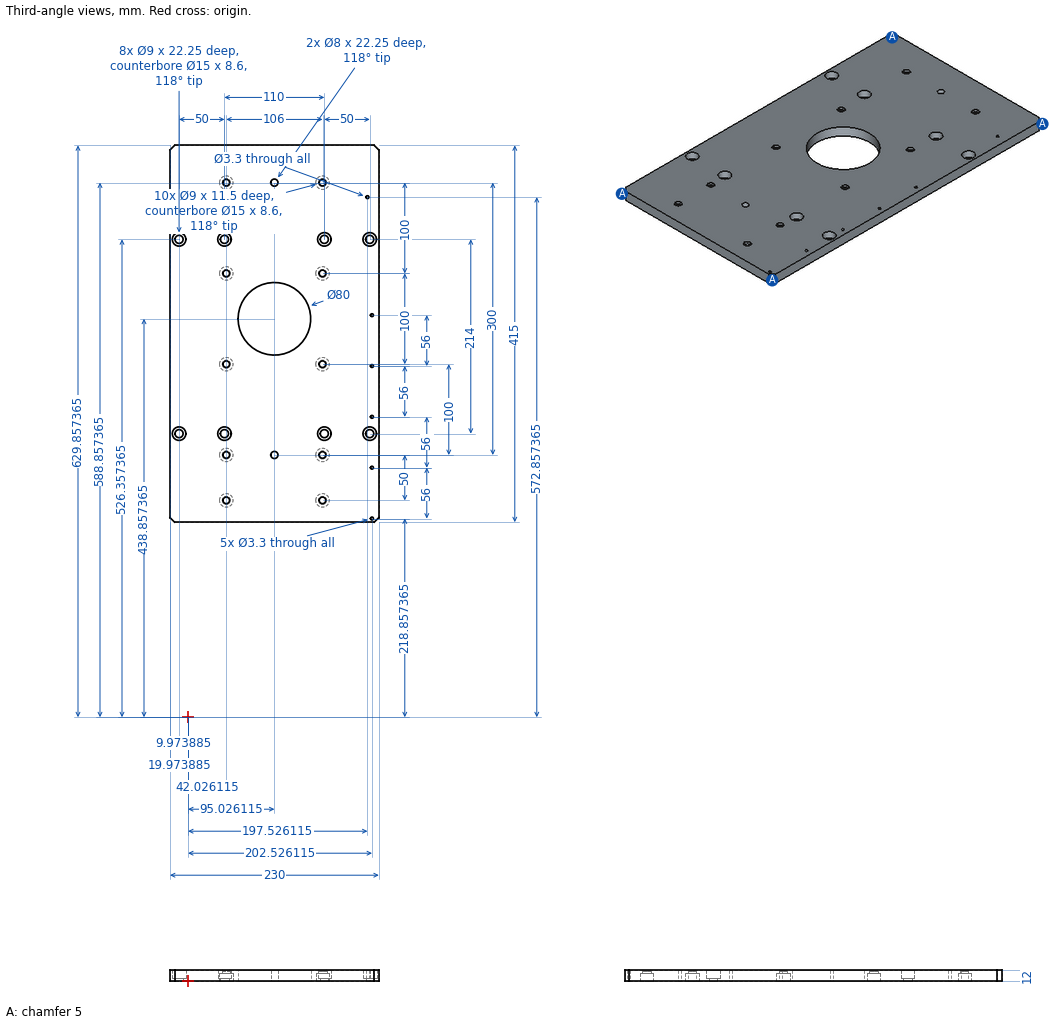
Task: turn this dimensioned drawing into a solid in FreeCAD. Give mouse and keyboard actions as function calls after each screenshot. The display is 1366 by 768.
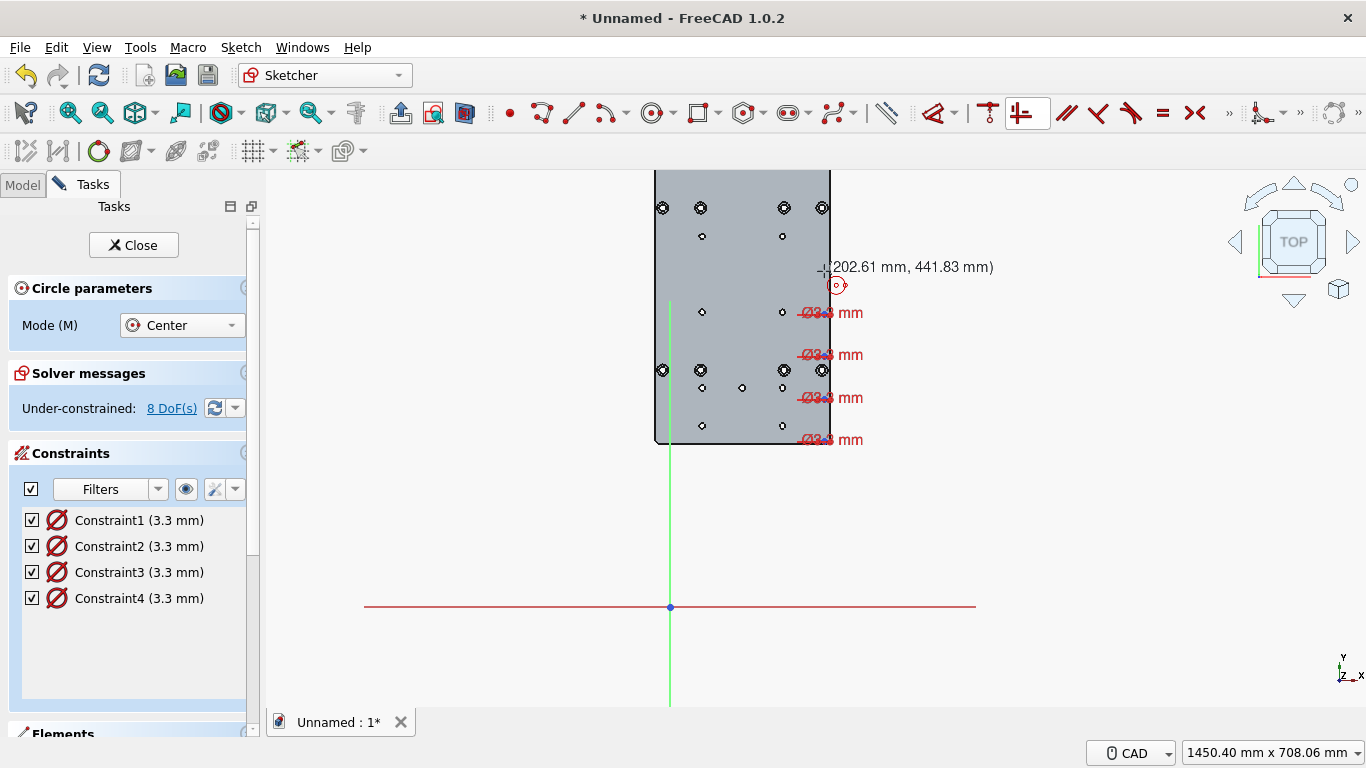
click(824, 271)
move(825, 270)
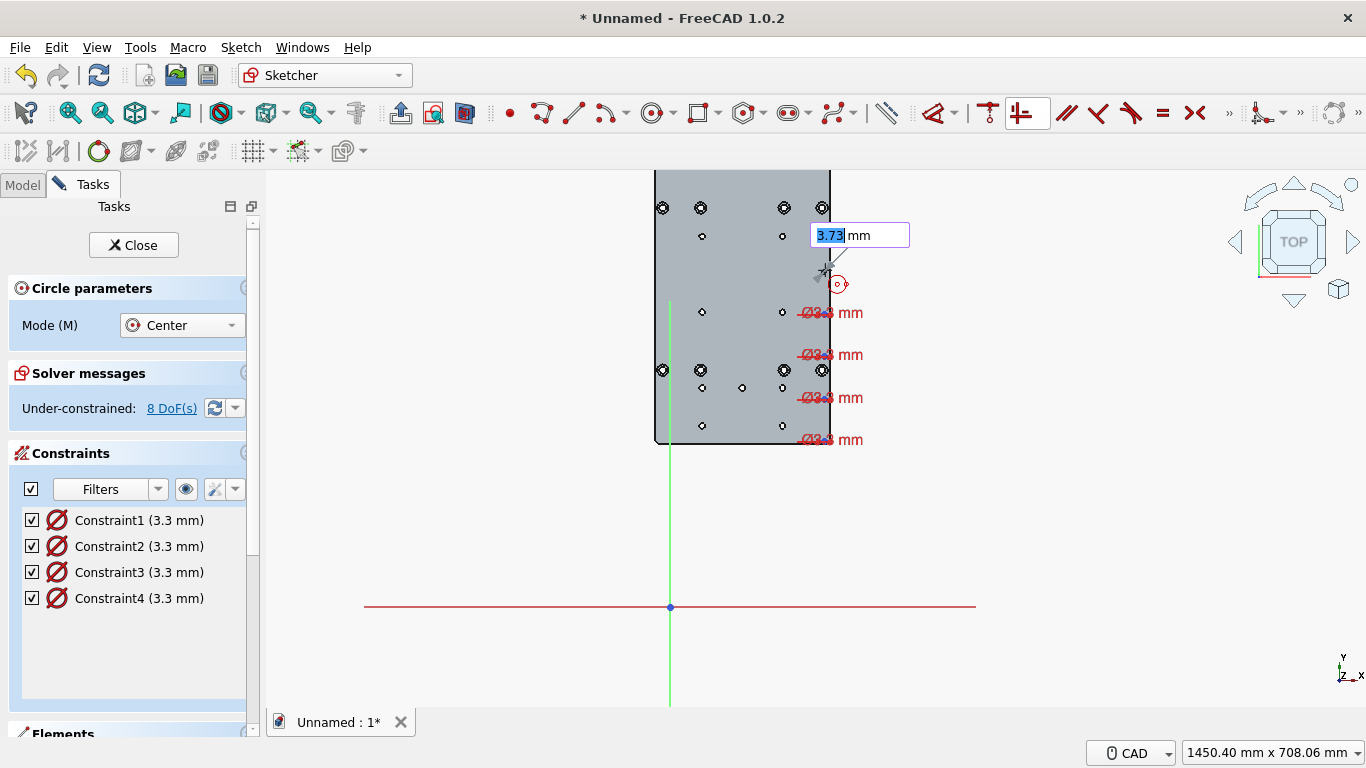
text(3.3)
key(Return)
key(Escape)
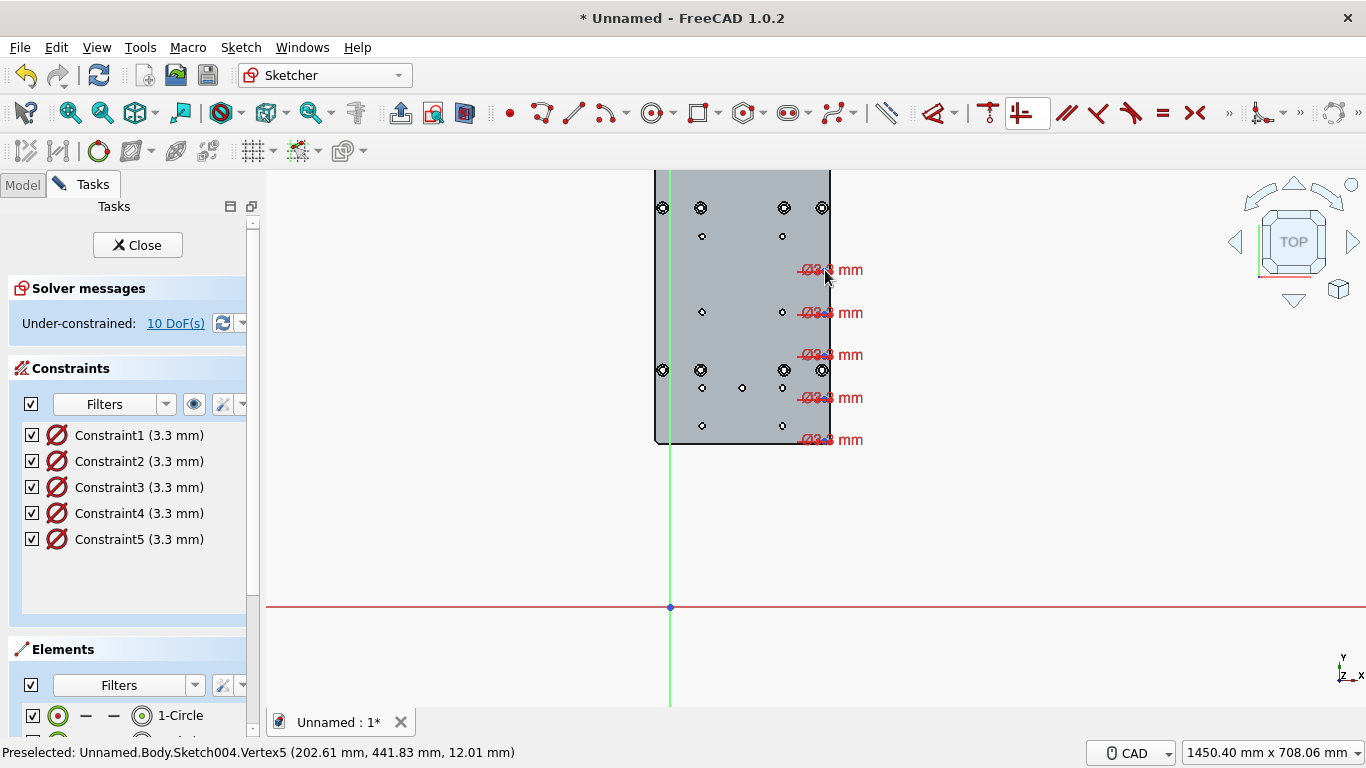
click(824, 442)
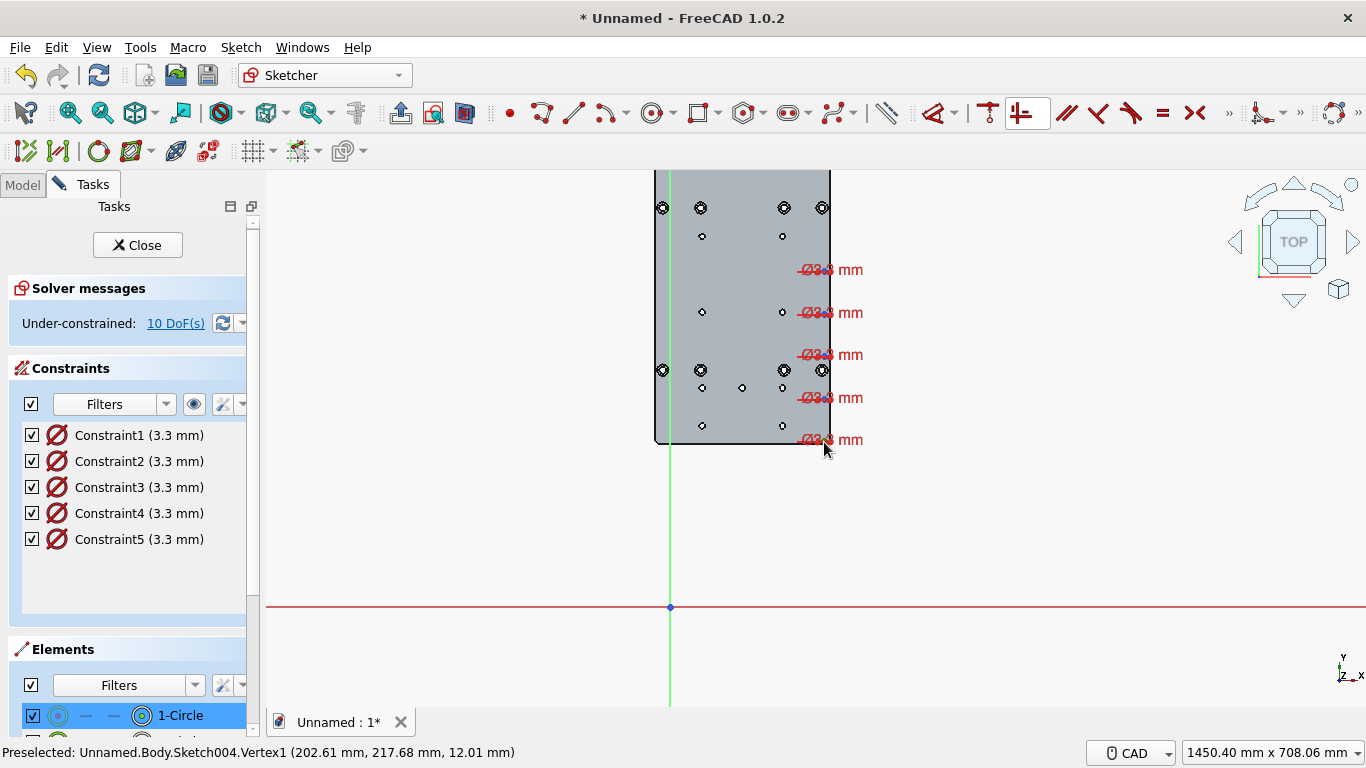
click(824, 400)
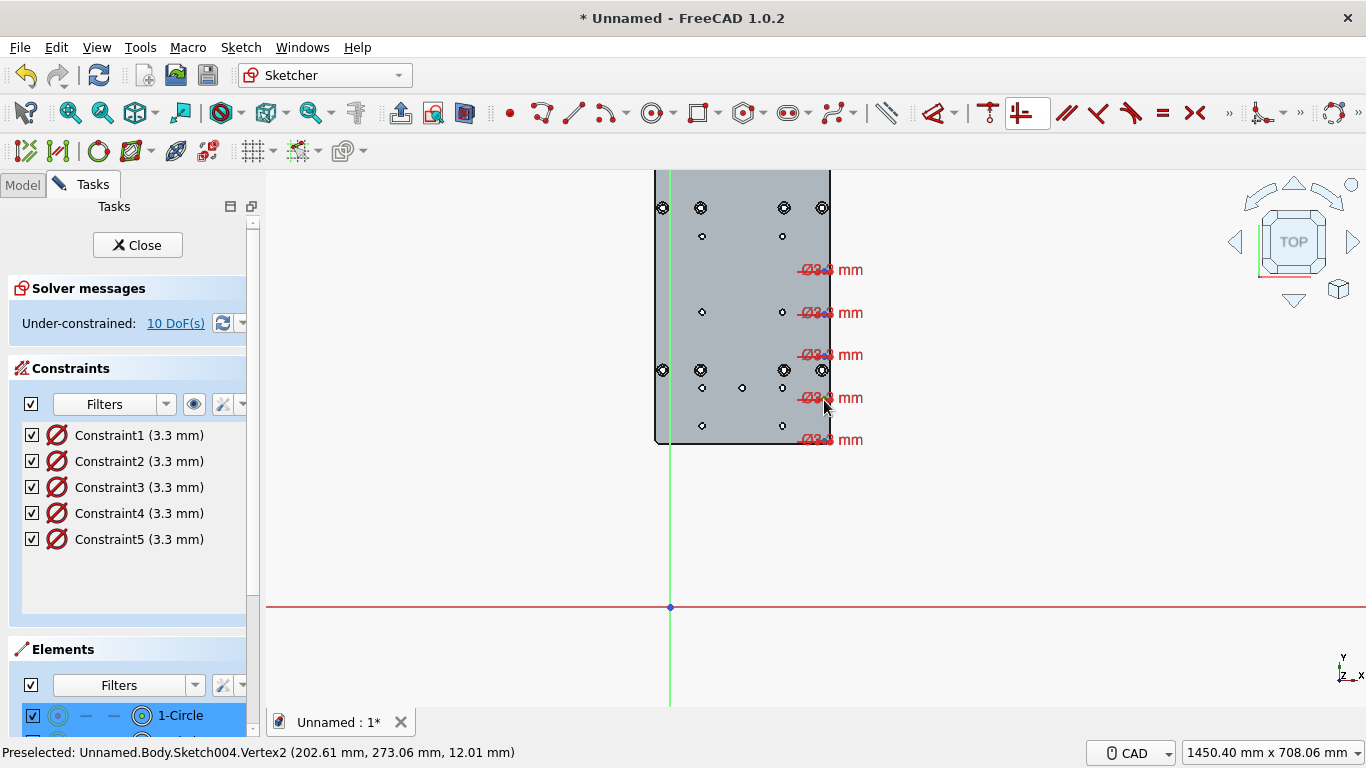
key(v)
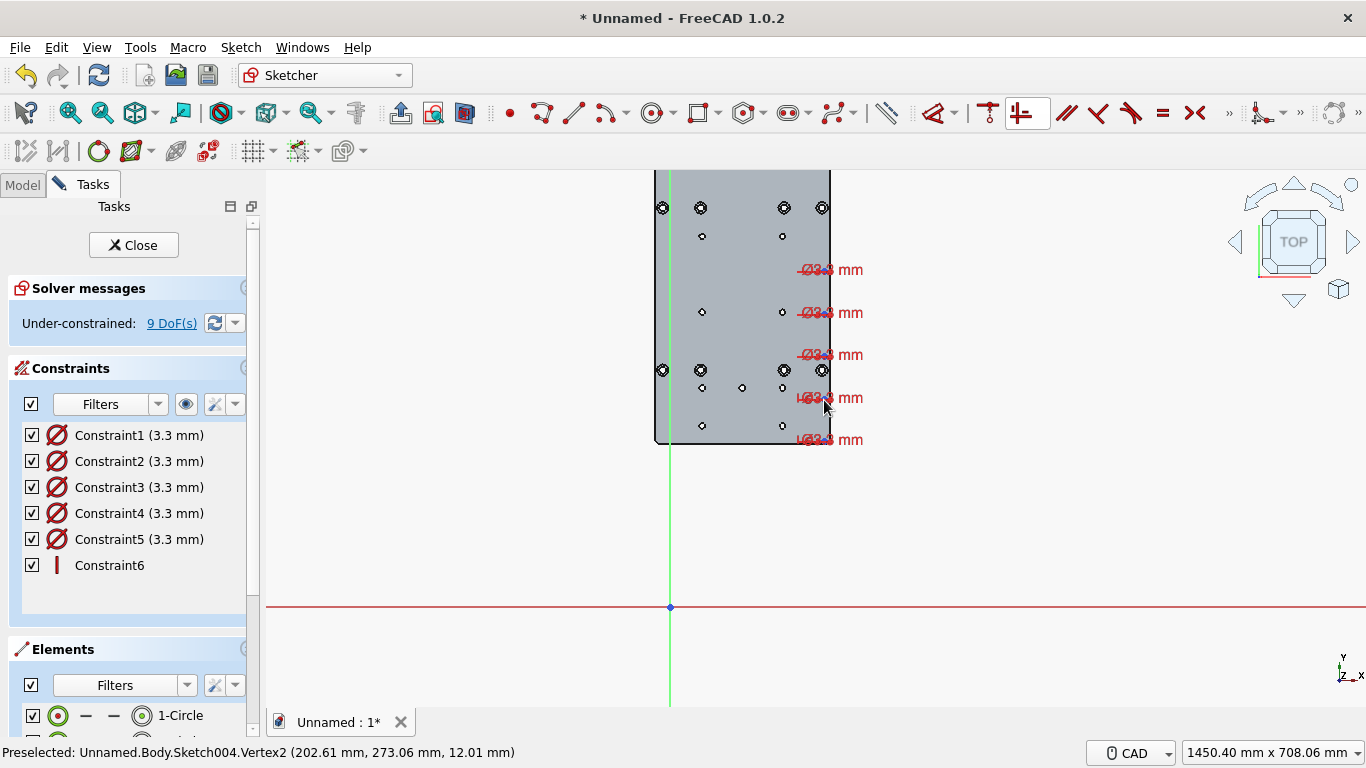
click(824, 400)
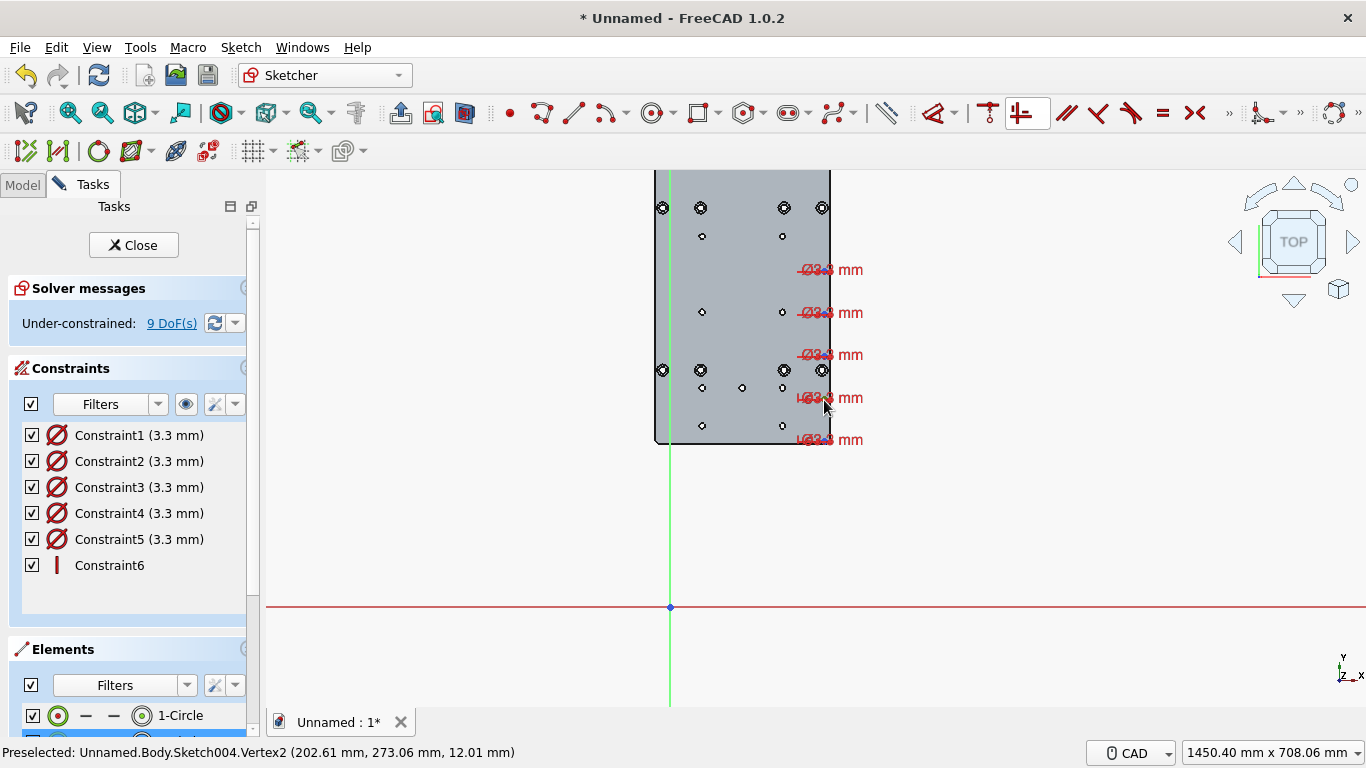
click(824, 357)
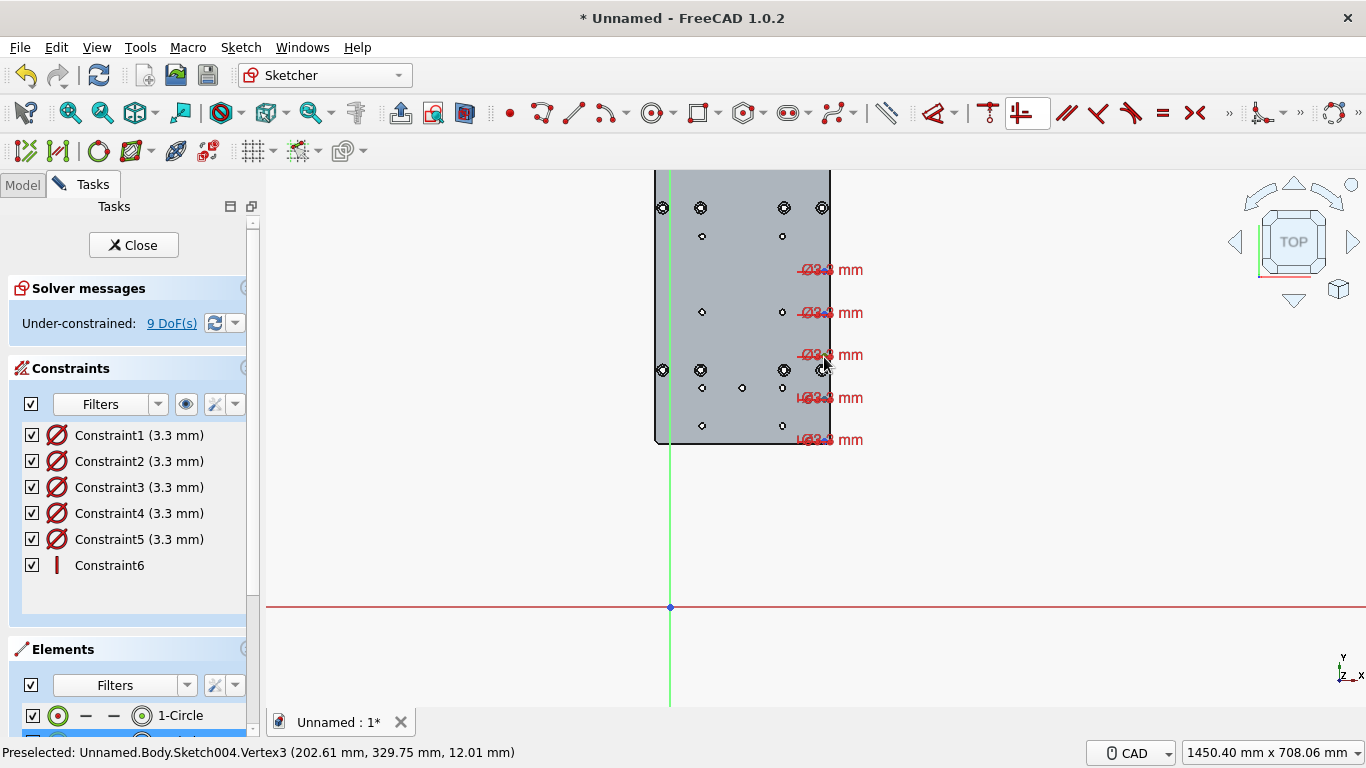
key(v)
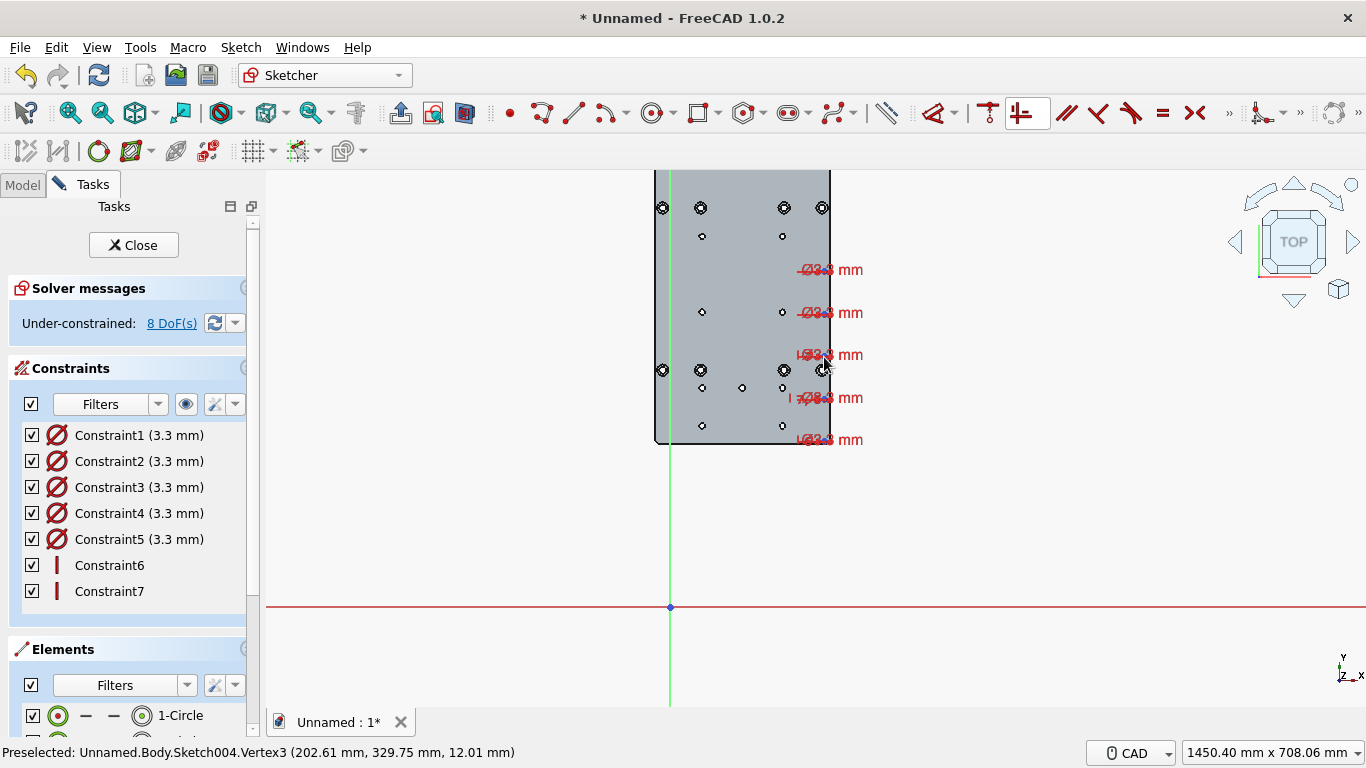
click(824, 357)